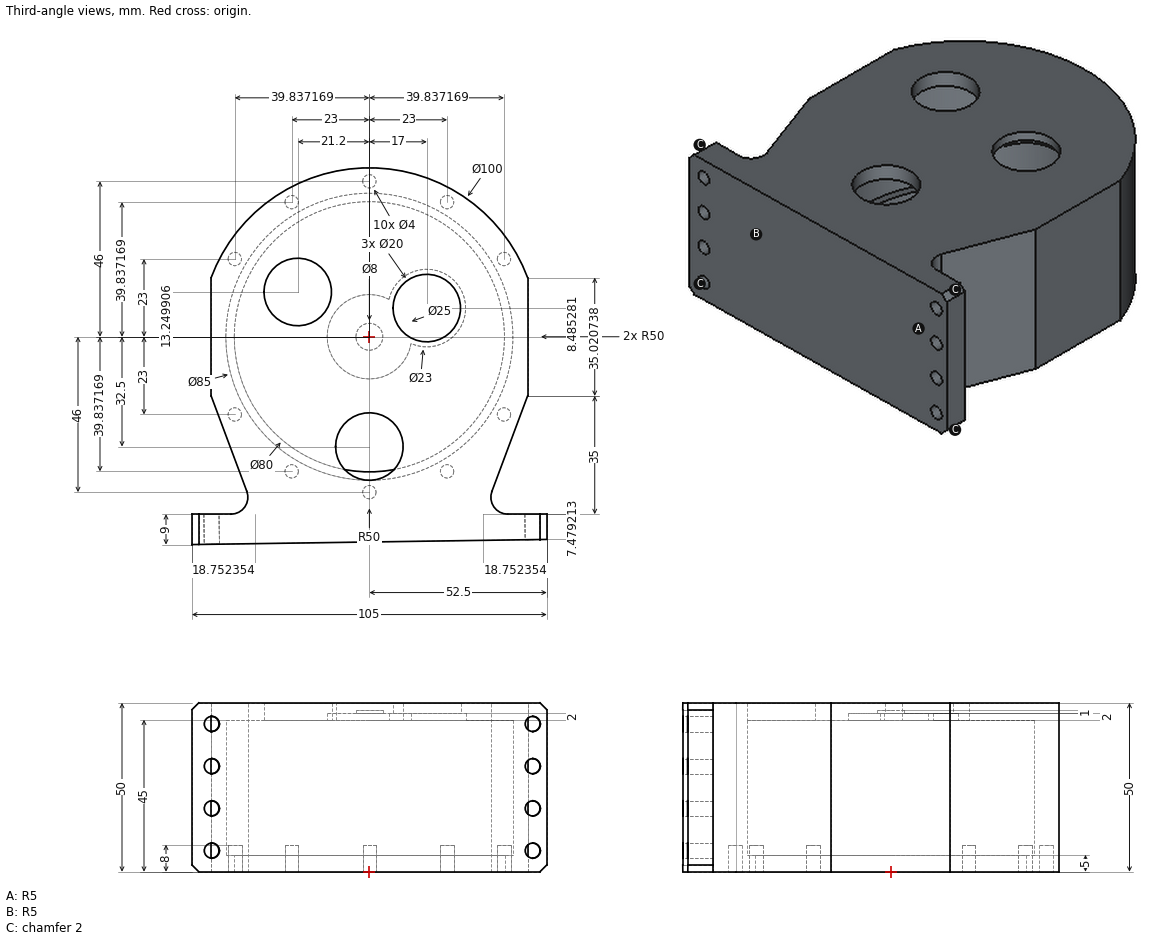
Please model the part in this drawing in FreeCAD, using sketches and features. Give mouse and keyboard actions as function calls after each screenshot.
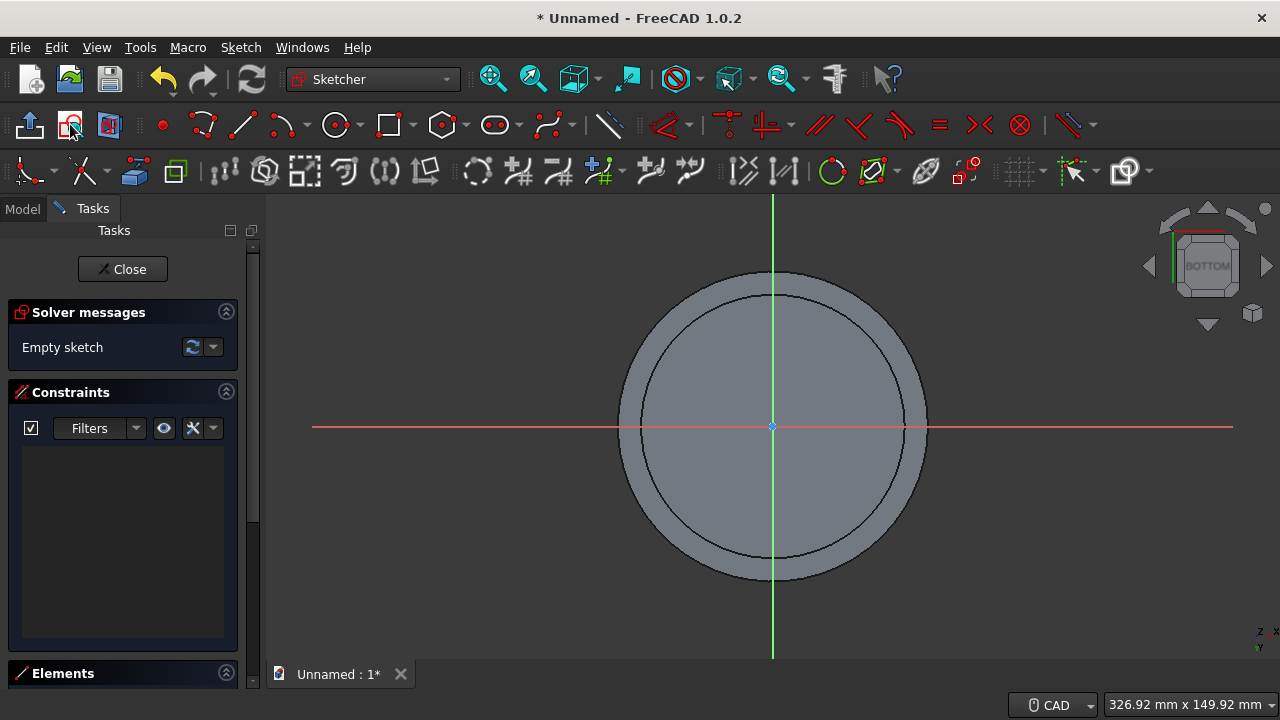
scroll(795, 426, up, 7)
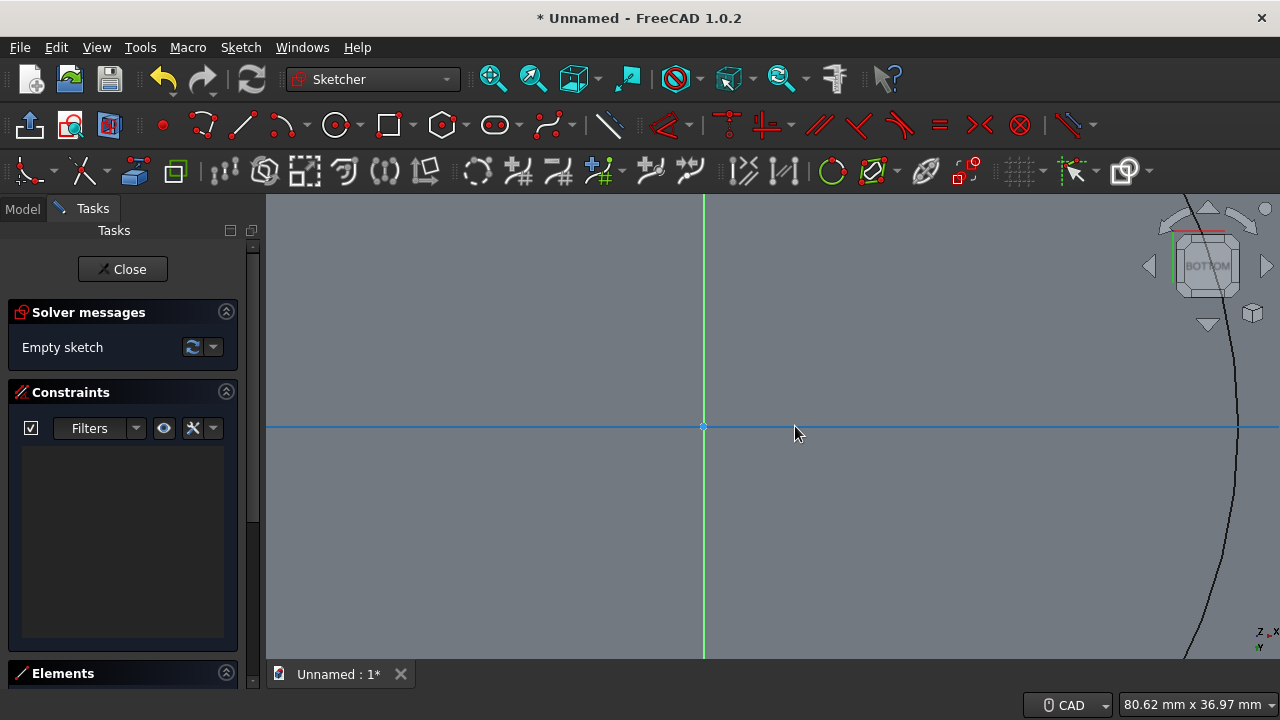
click(336, 126)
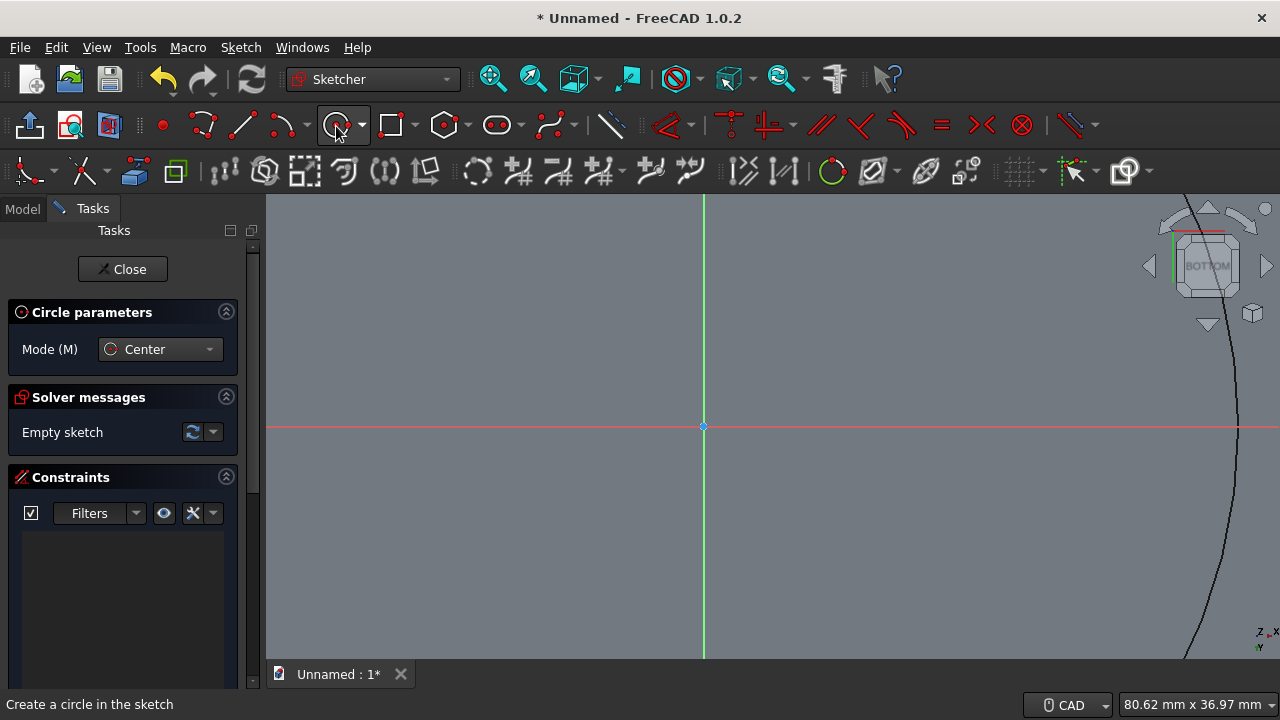
click(704, 426)
click(815, 315)
key(Escape)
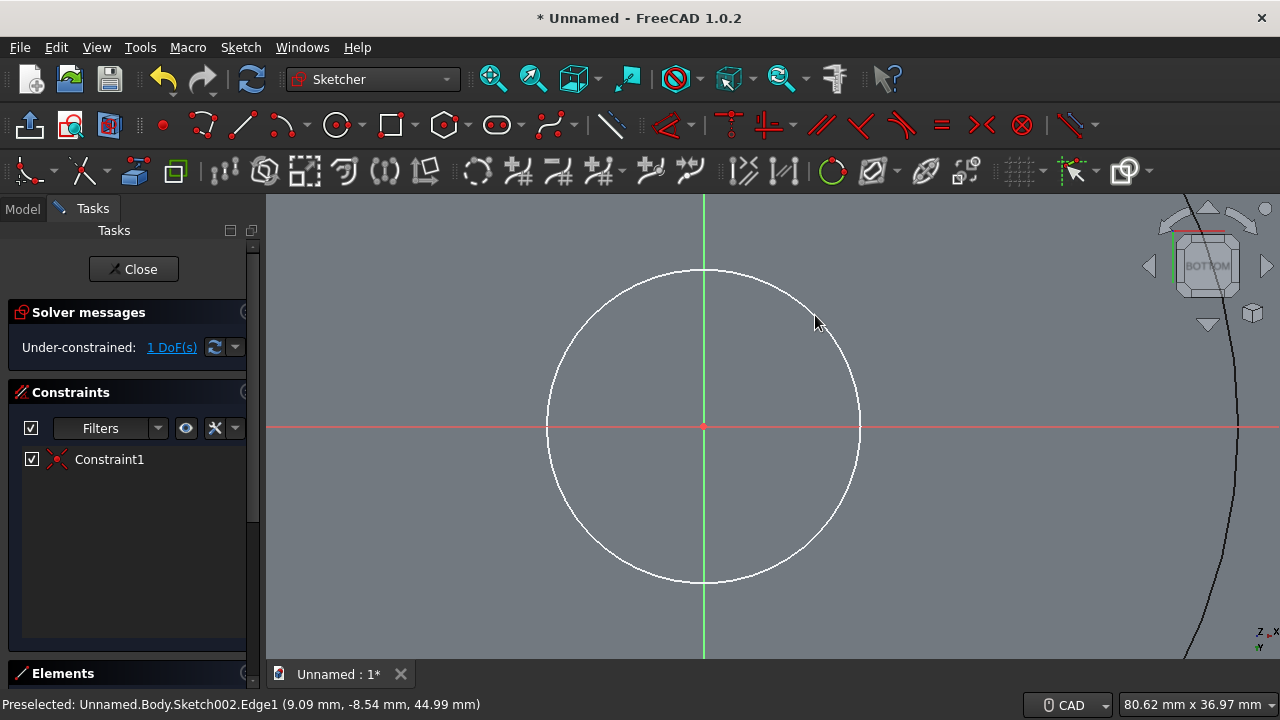
click(666, 126)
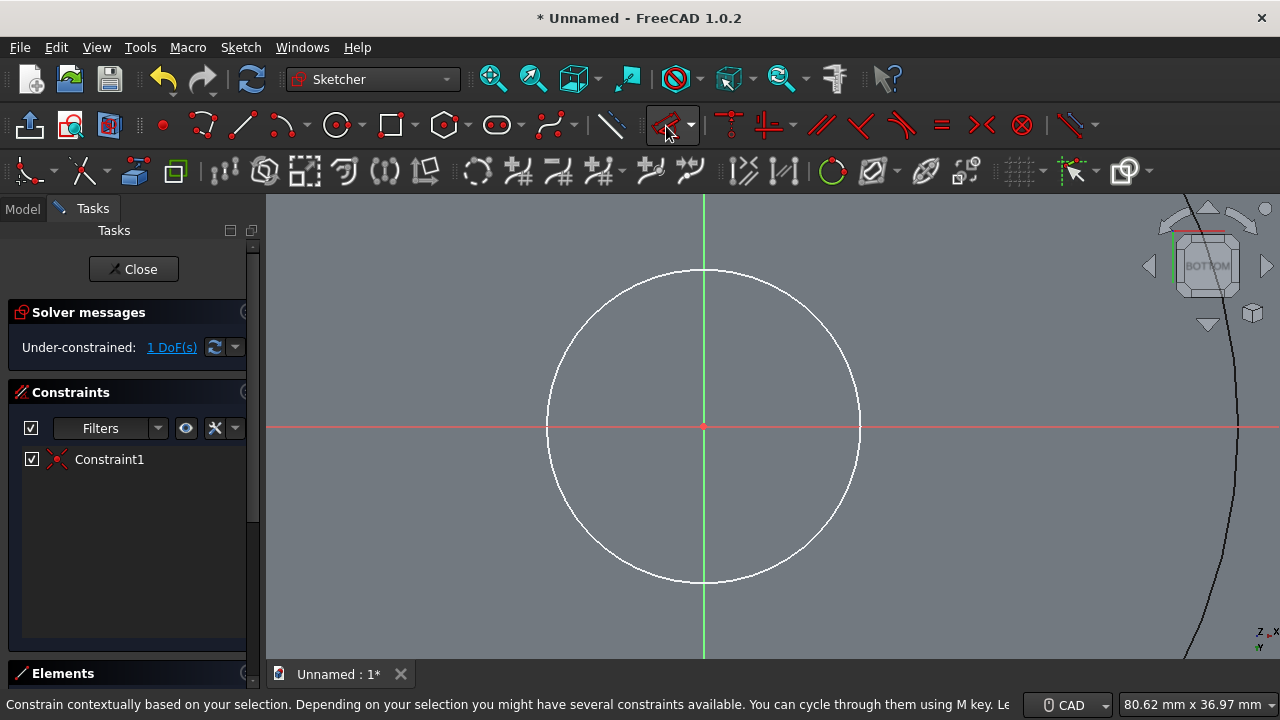
click(814, 315)
click(837, 292)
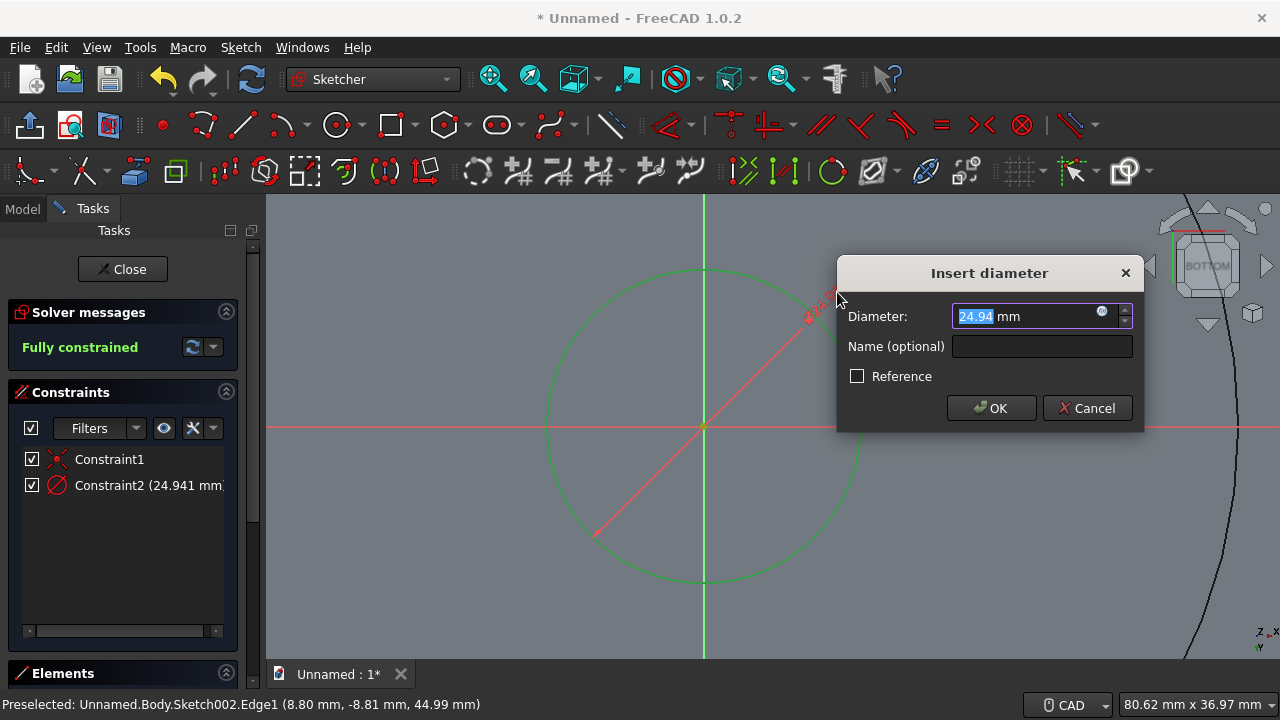
text(25)
key(Return)
key(Escape)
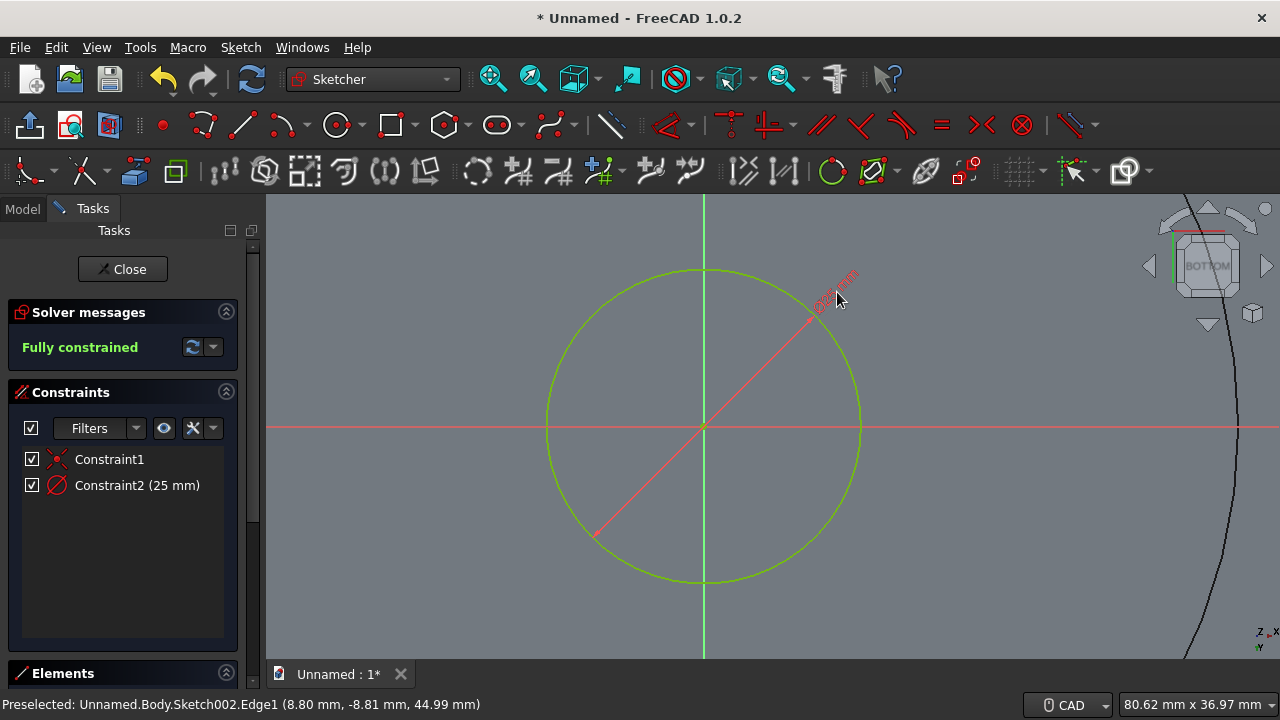
click(123, 269)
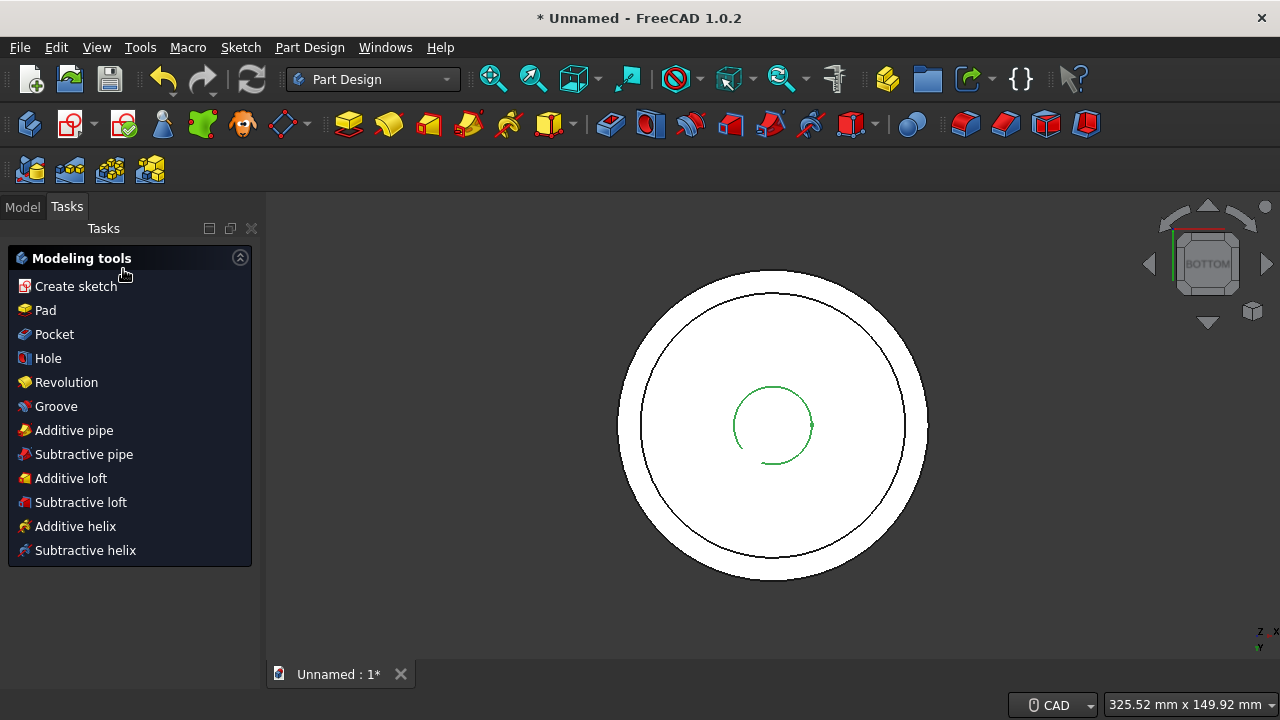
click(612, 124)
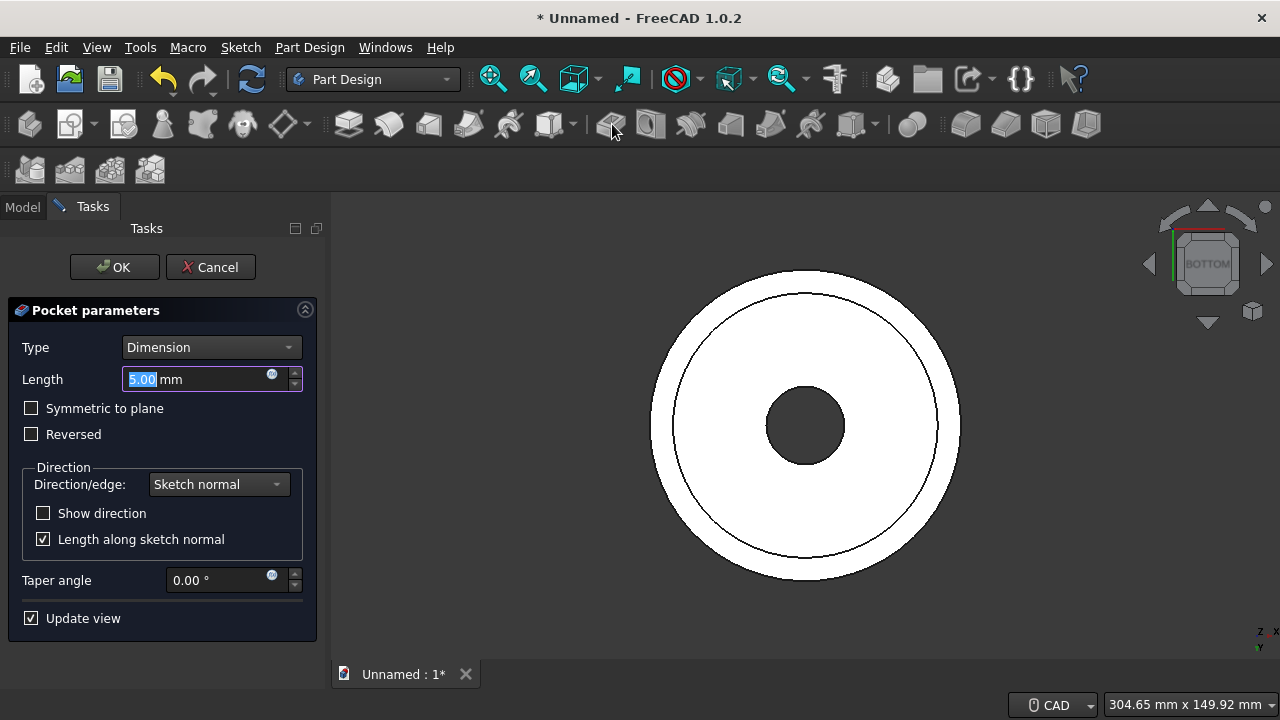
text(2)
key(Tab)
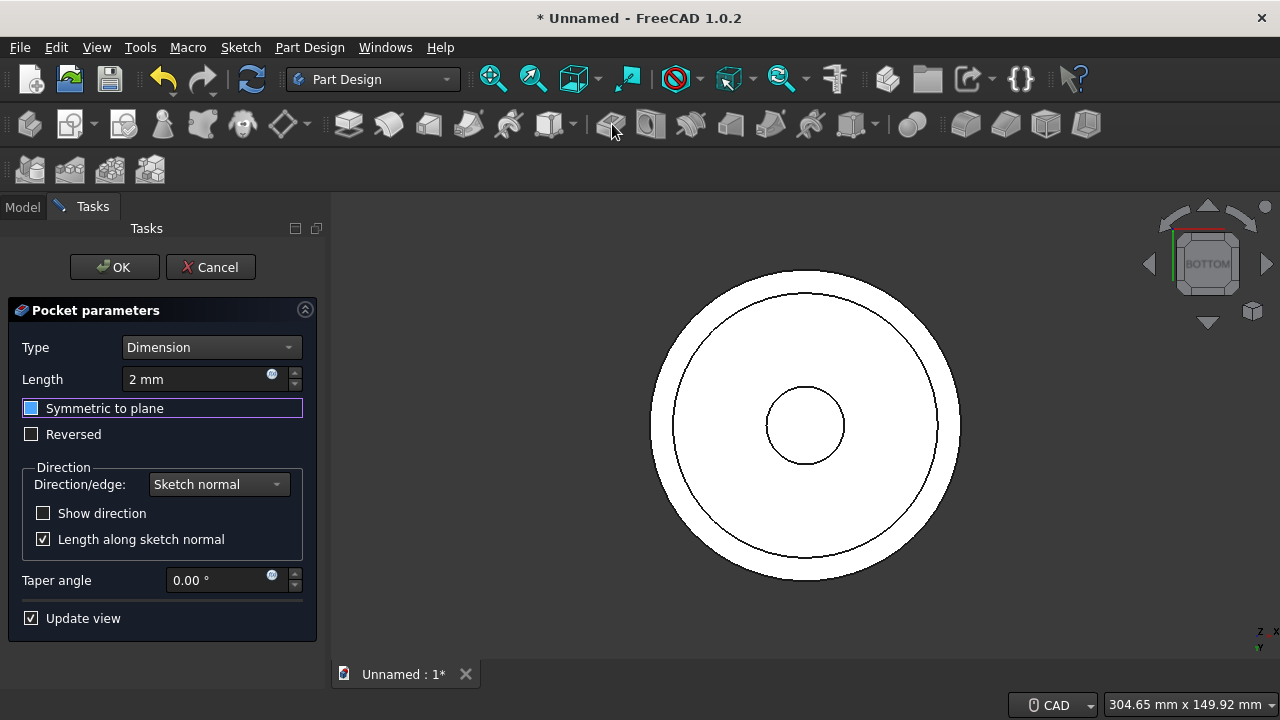
click(115, 267)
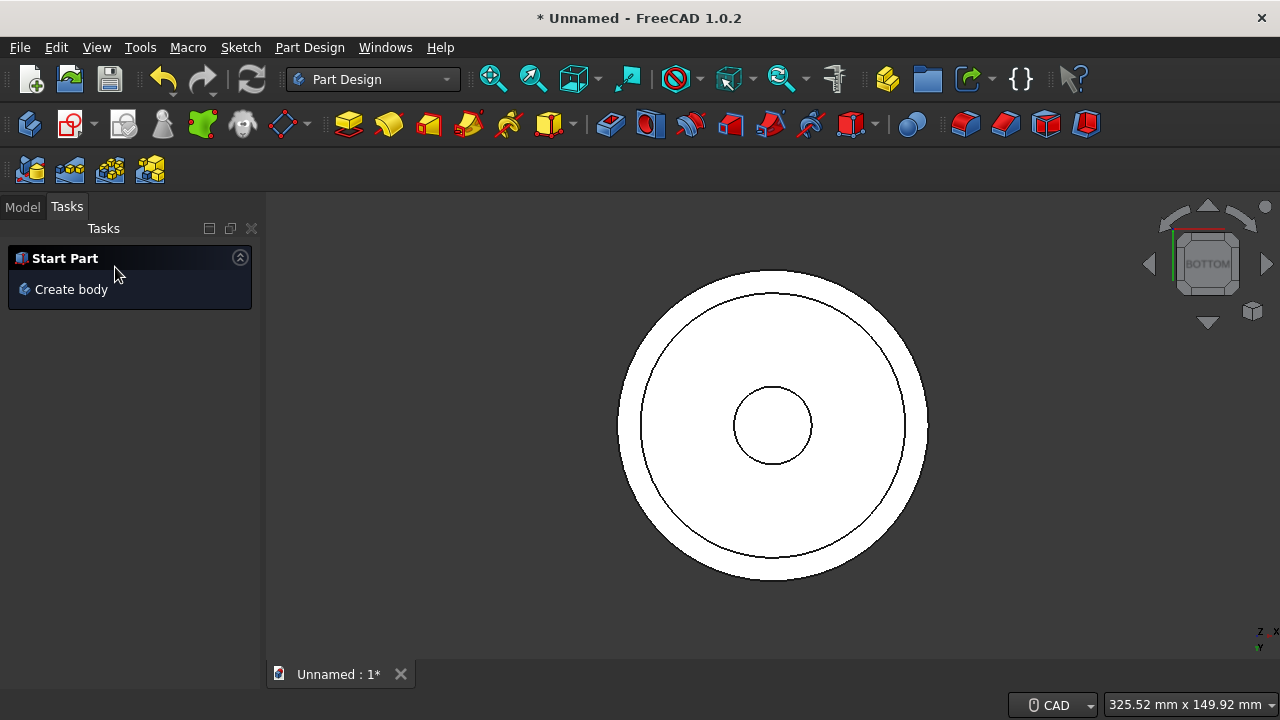
click(735, 500)